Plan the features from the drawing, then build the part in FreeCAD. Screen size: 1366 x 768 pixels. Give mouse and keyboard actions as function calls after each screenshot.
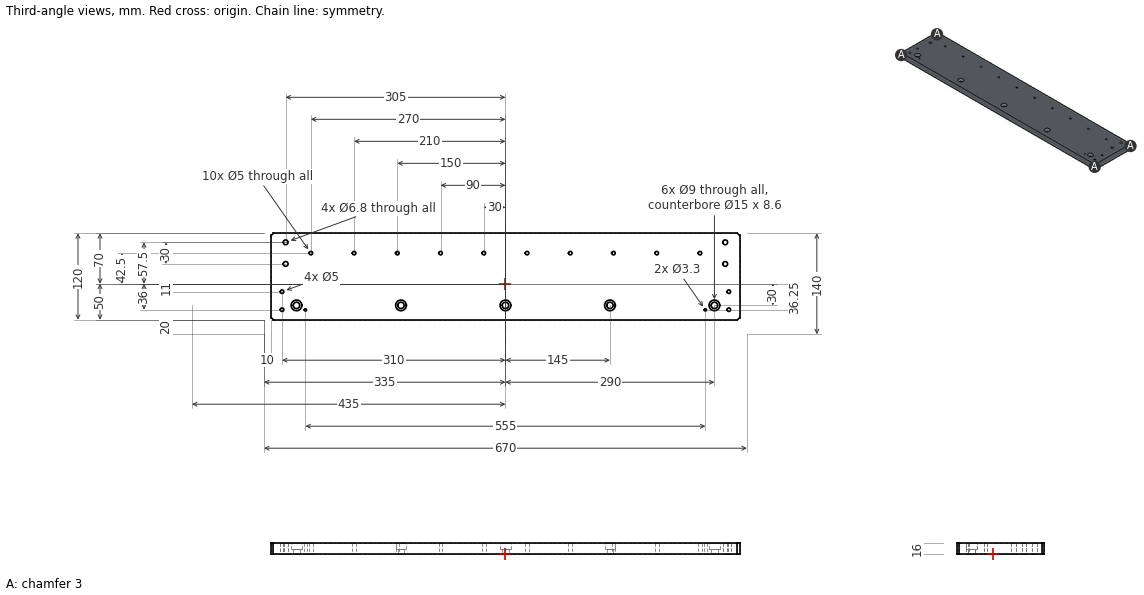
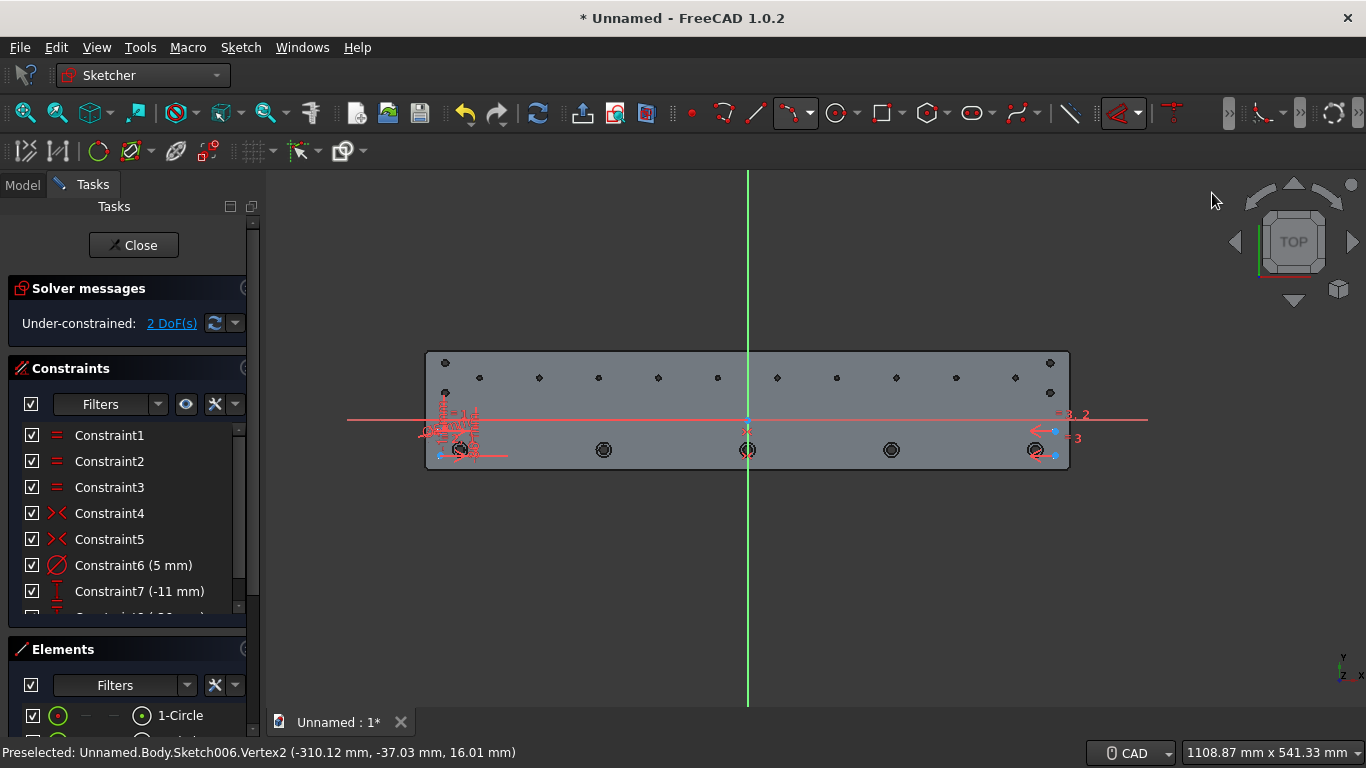
click(440, 431)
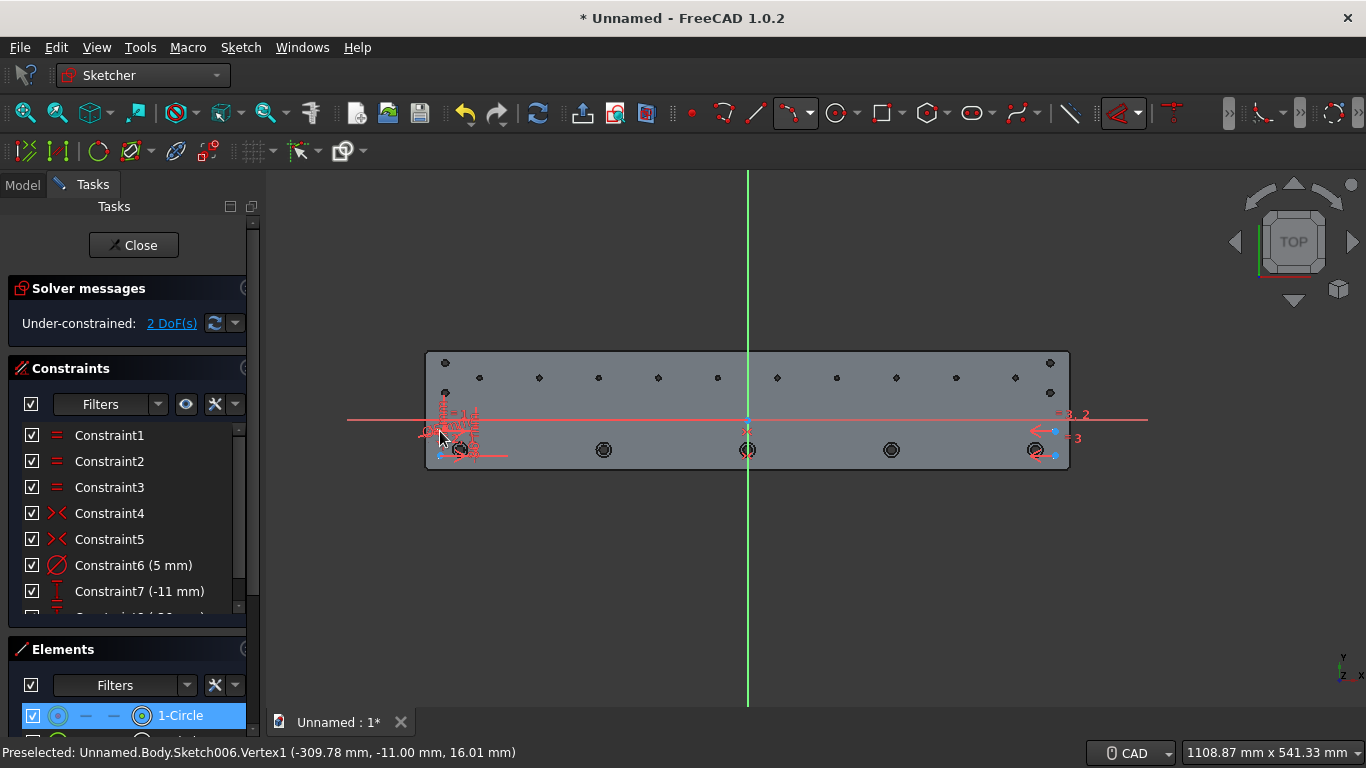
key(l)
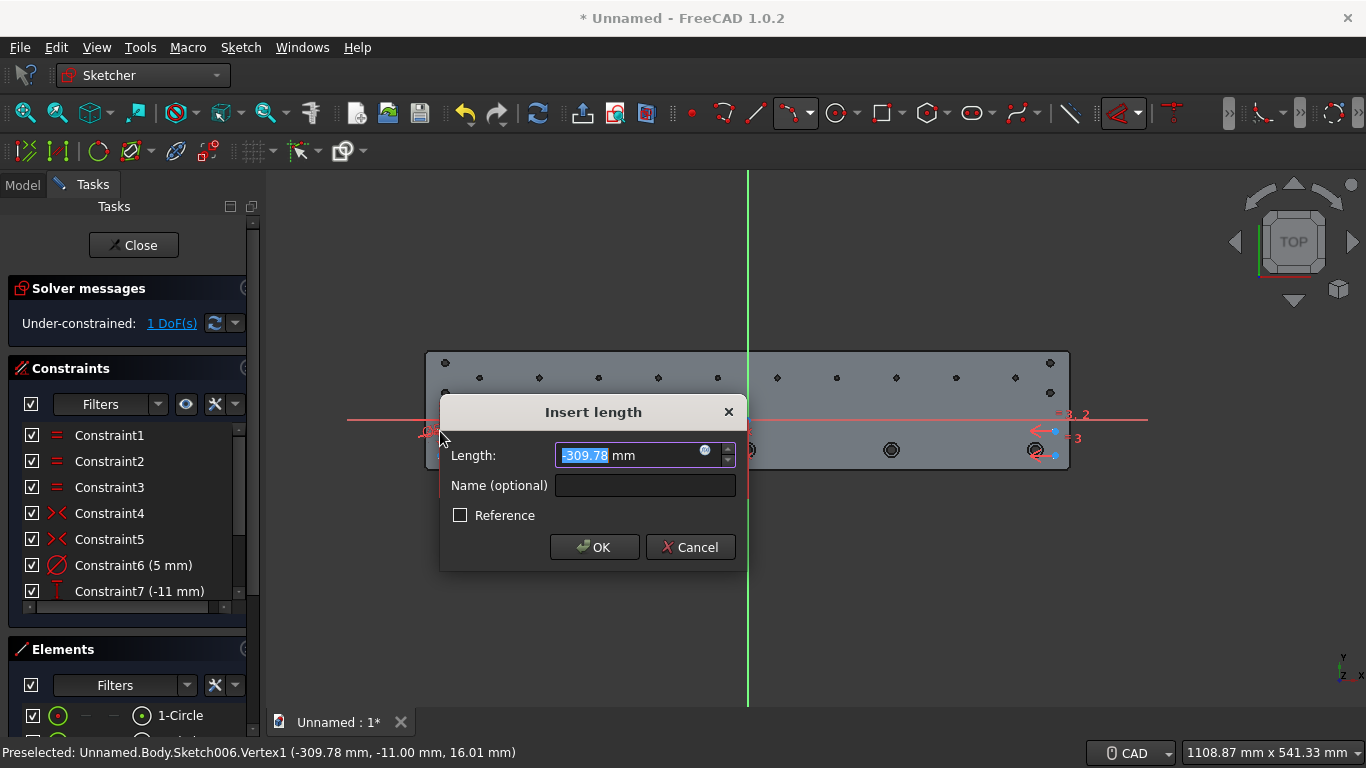
text(-310)
key(Return)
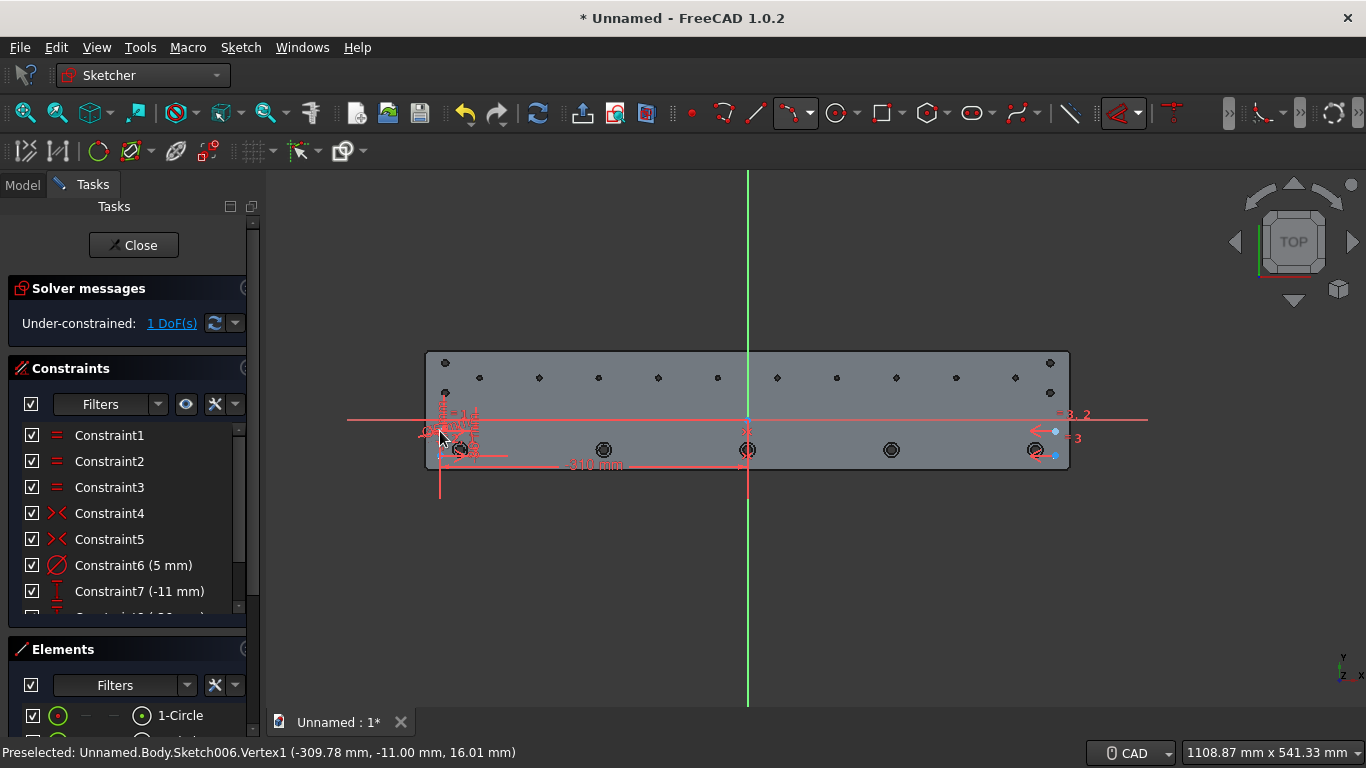
click(440, 456)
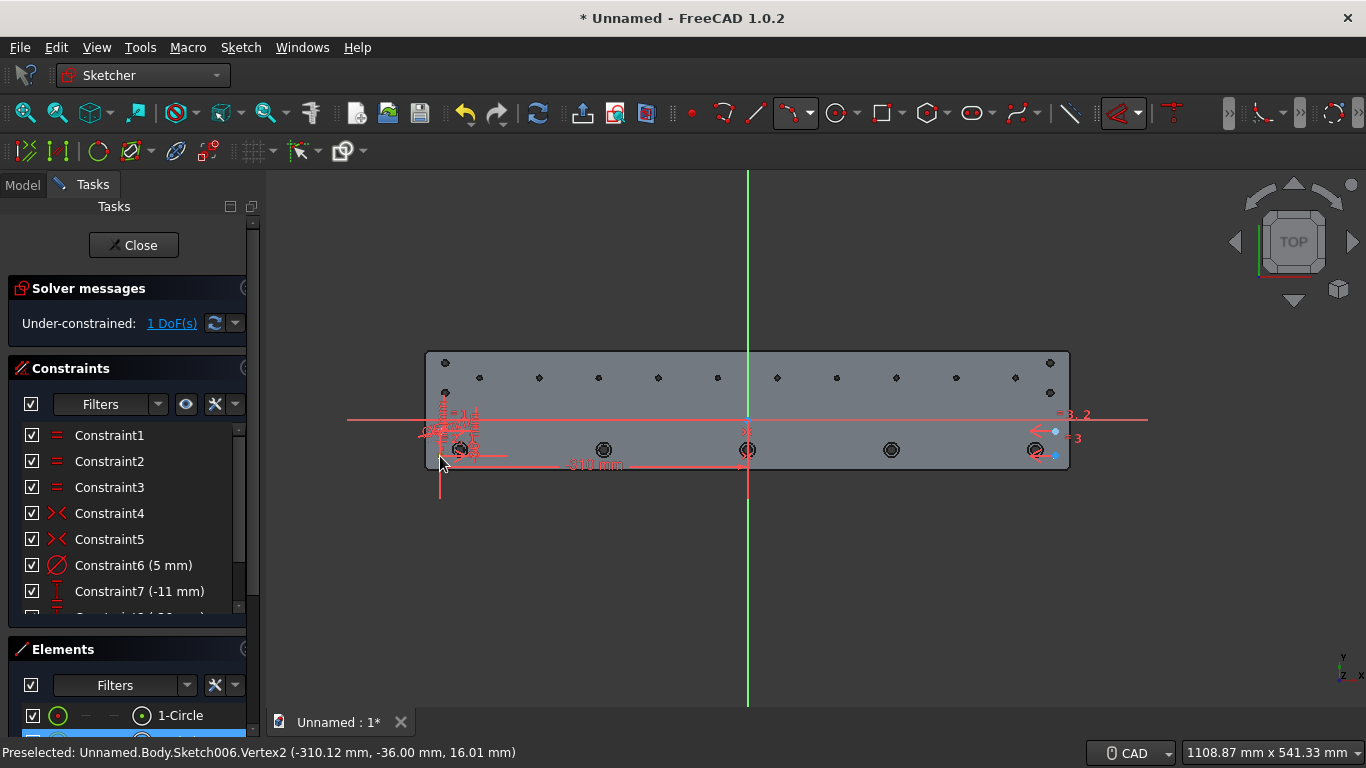
click(1140, 114)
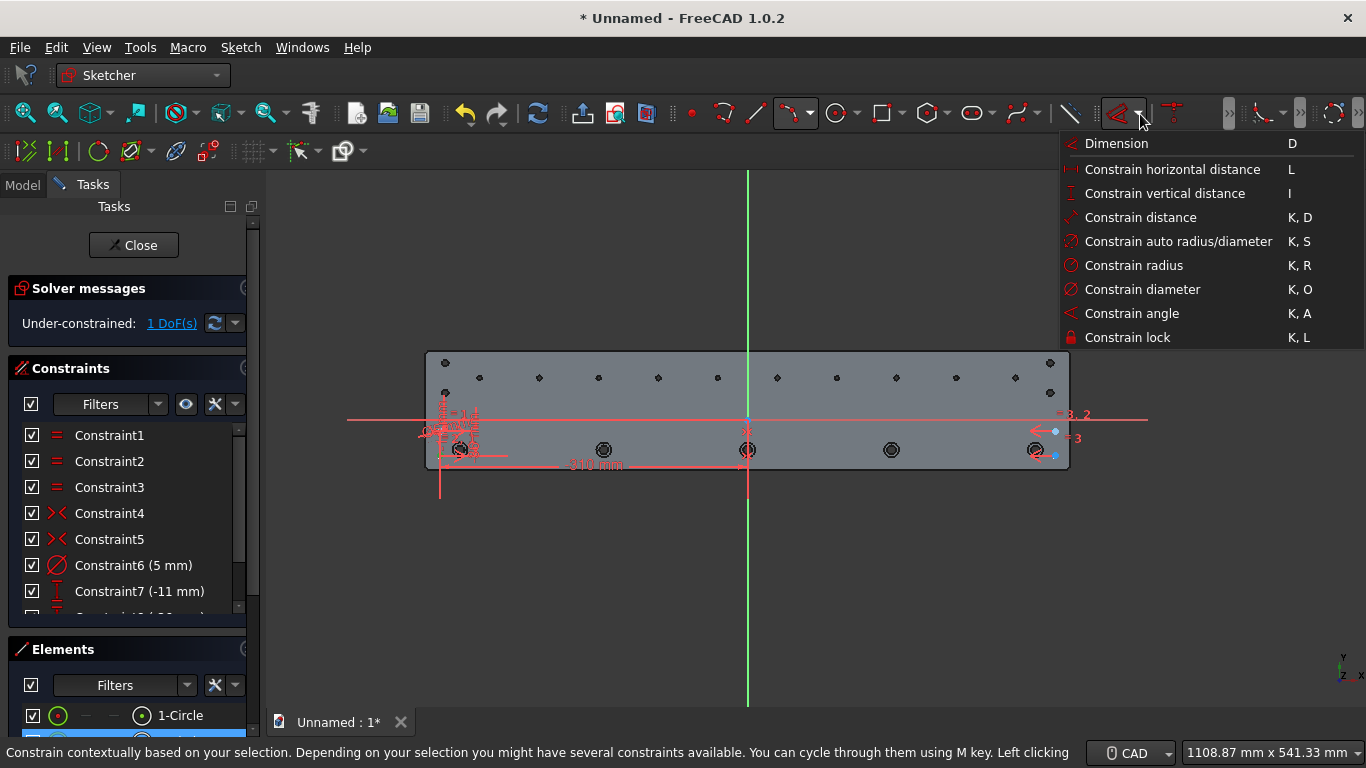
click(1212, 169)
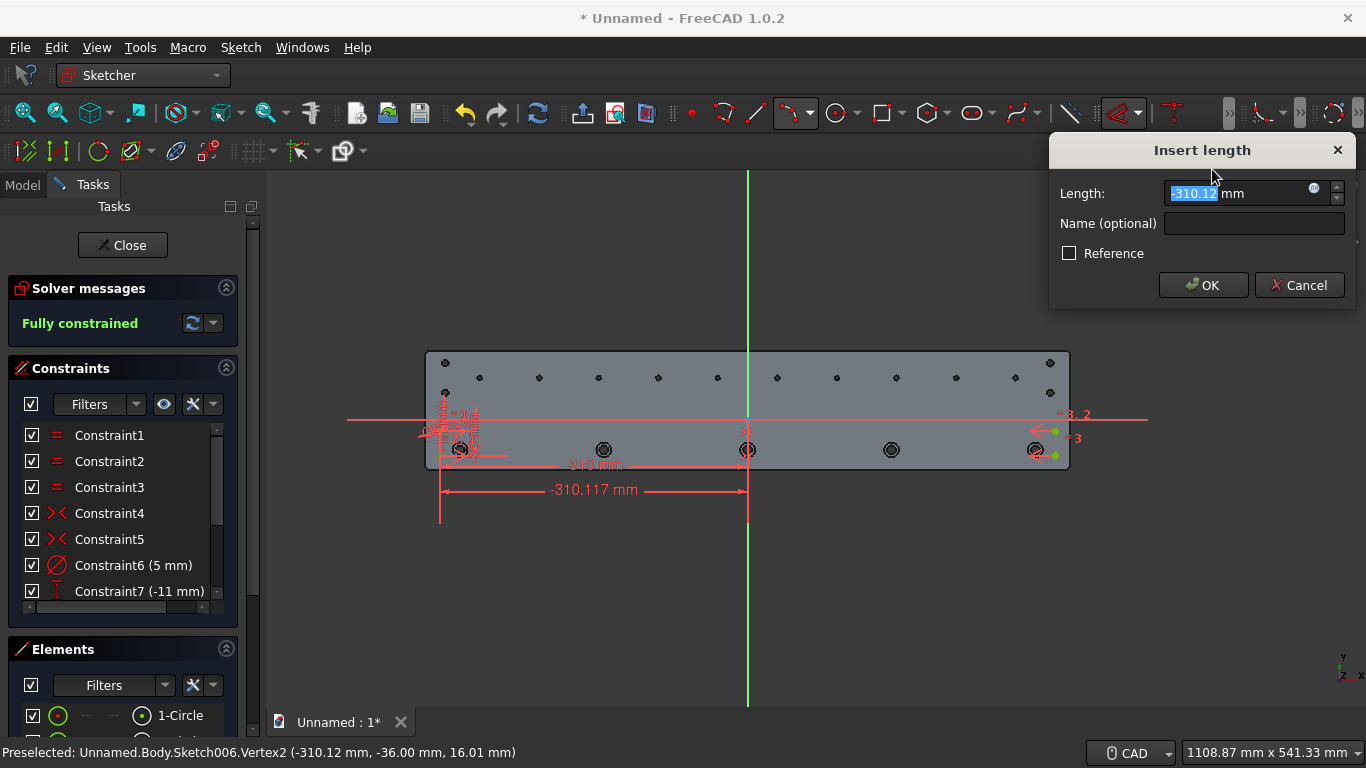
text(-310)
key(Return)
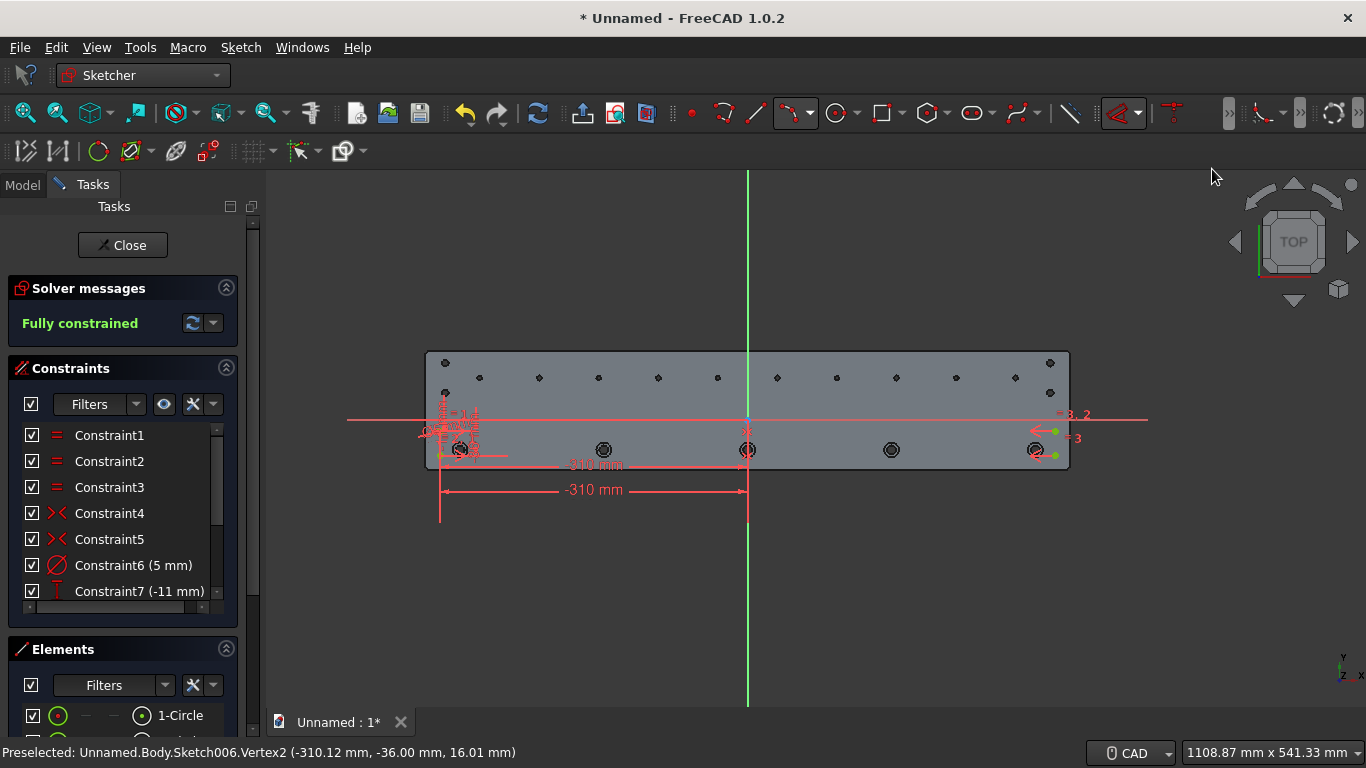
click(123, 245)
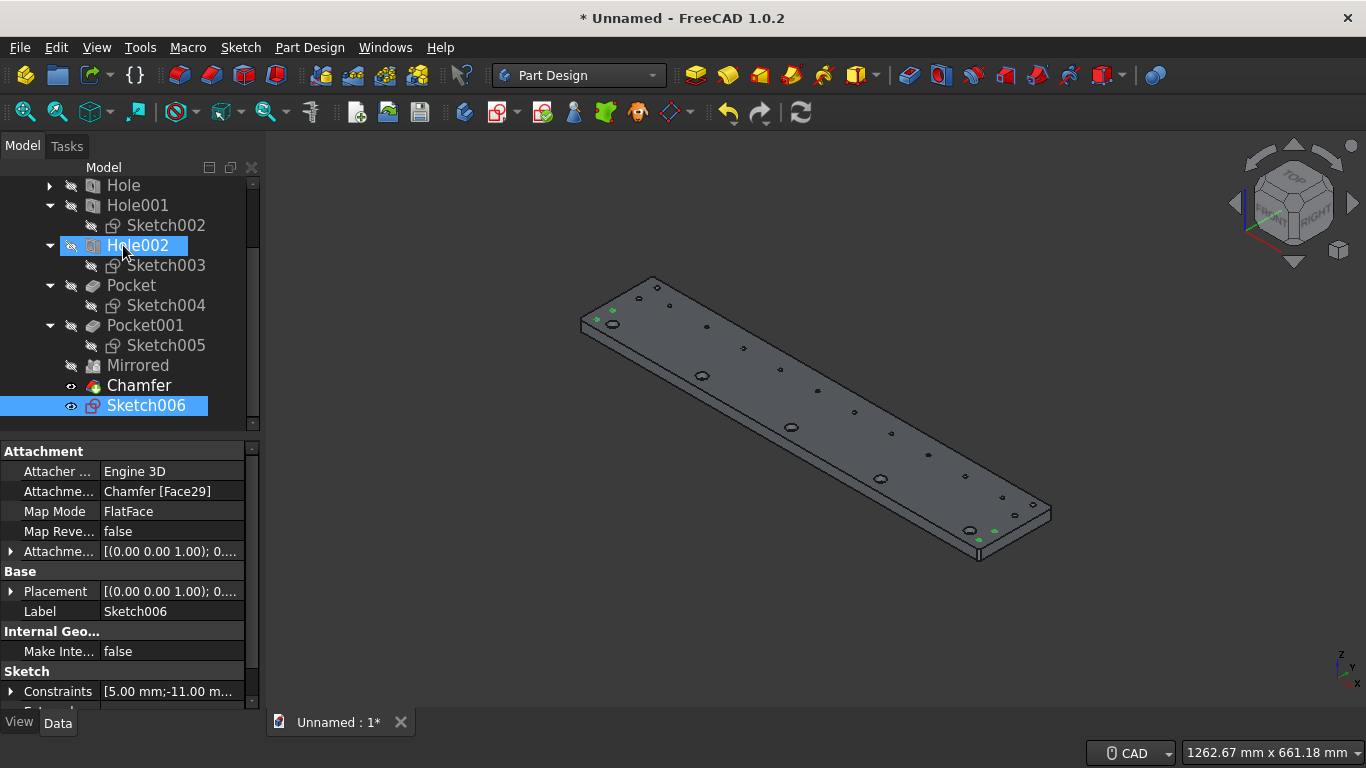
click(910, 76)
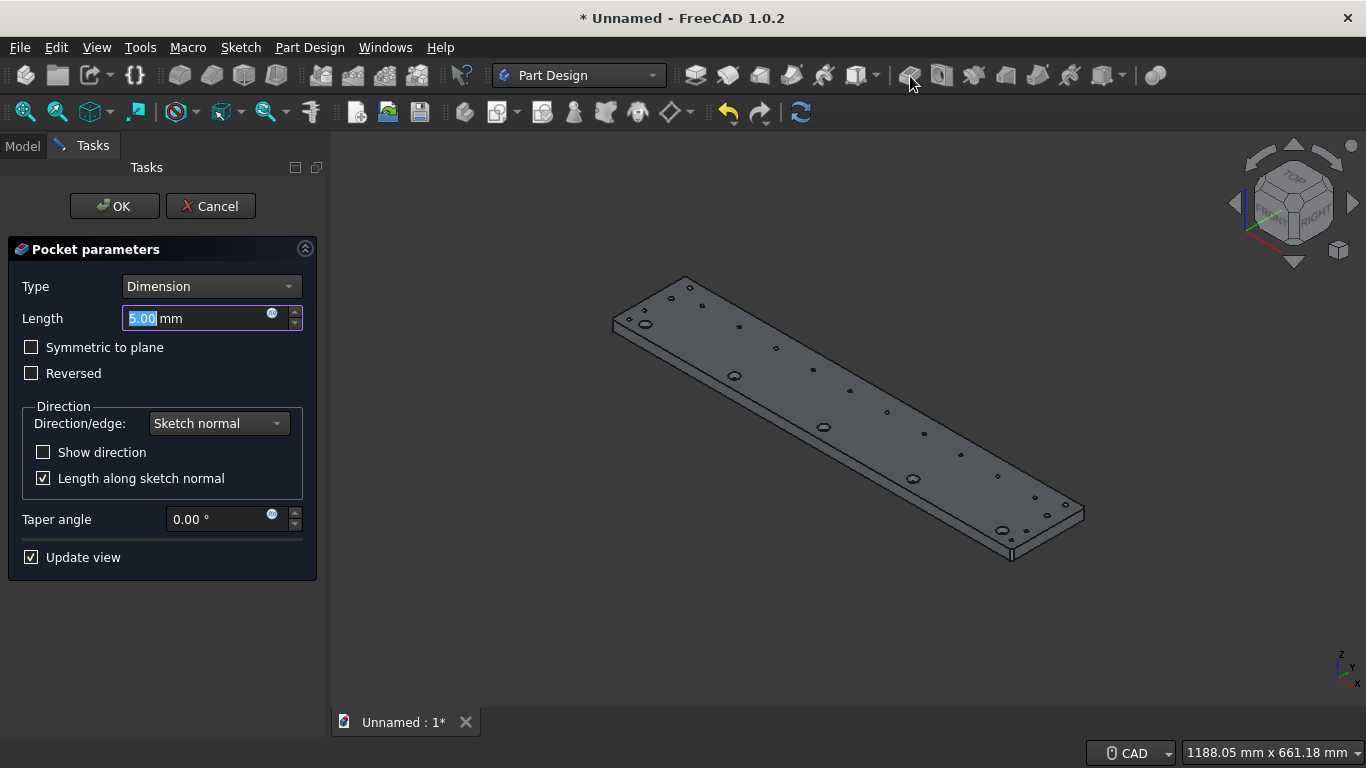
click(212, 286)